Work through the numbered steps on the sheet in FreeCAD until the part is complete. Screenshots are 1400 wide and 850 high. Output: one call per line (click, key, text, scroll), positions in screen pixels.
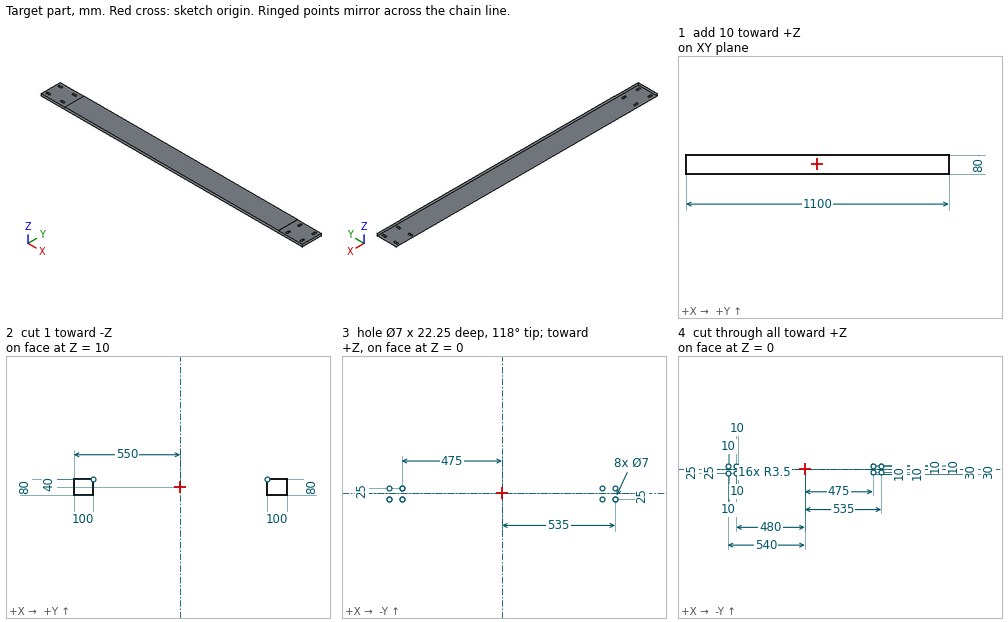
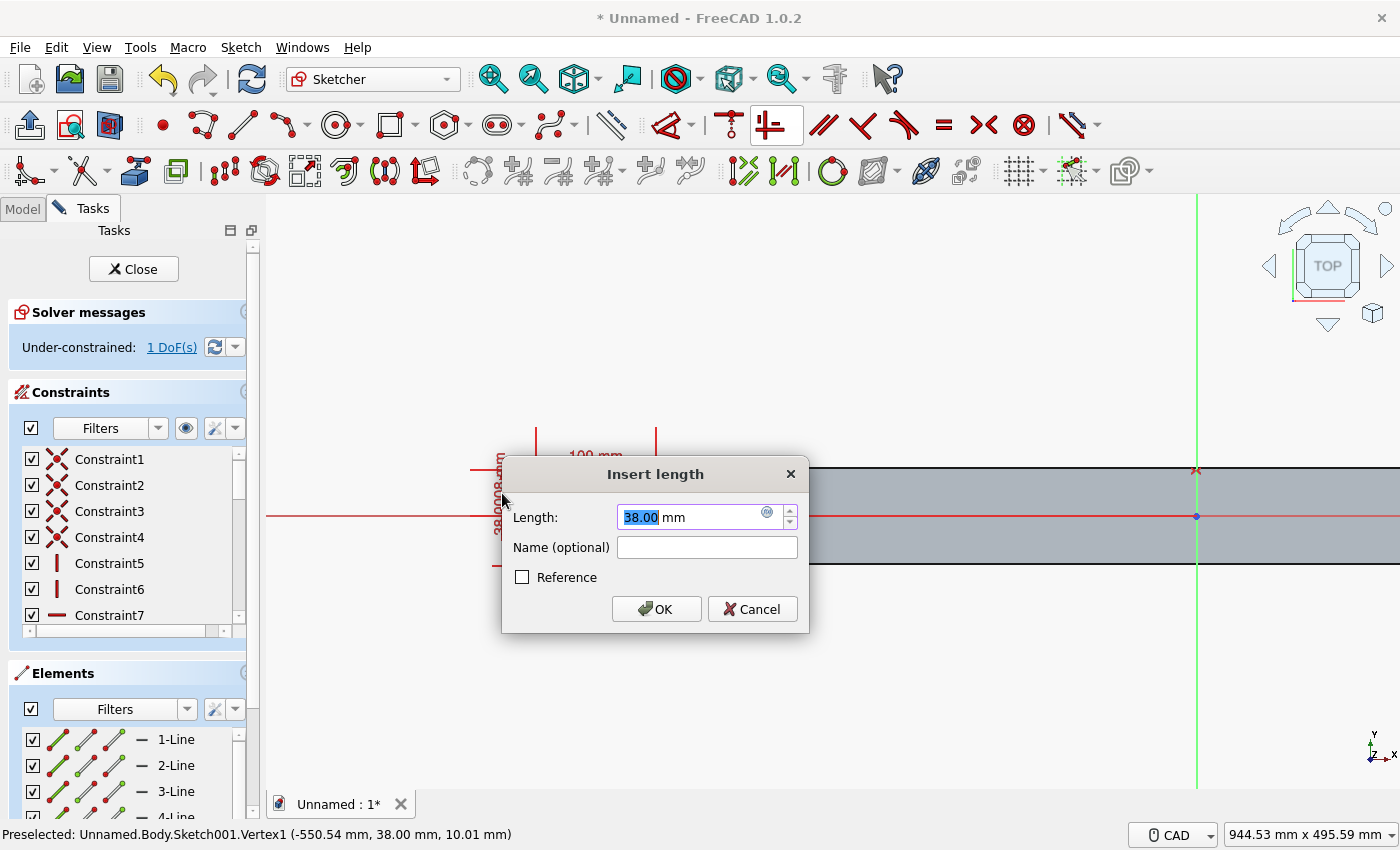
text(40)
key(Return)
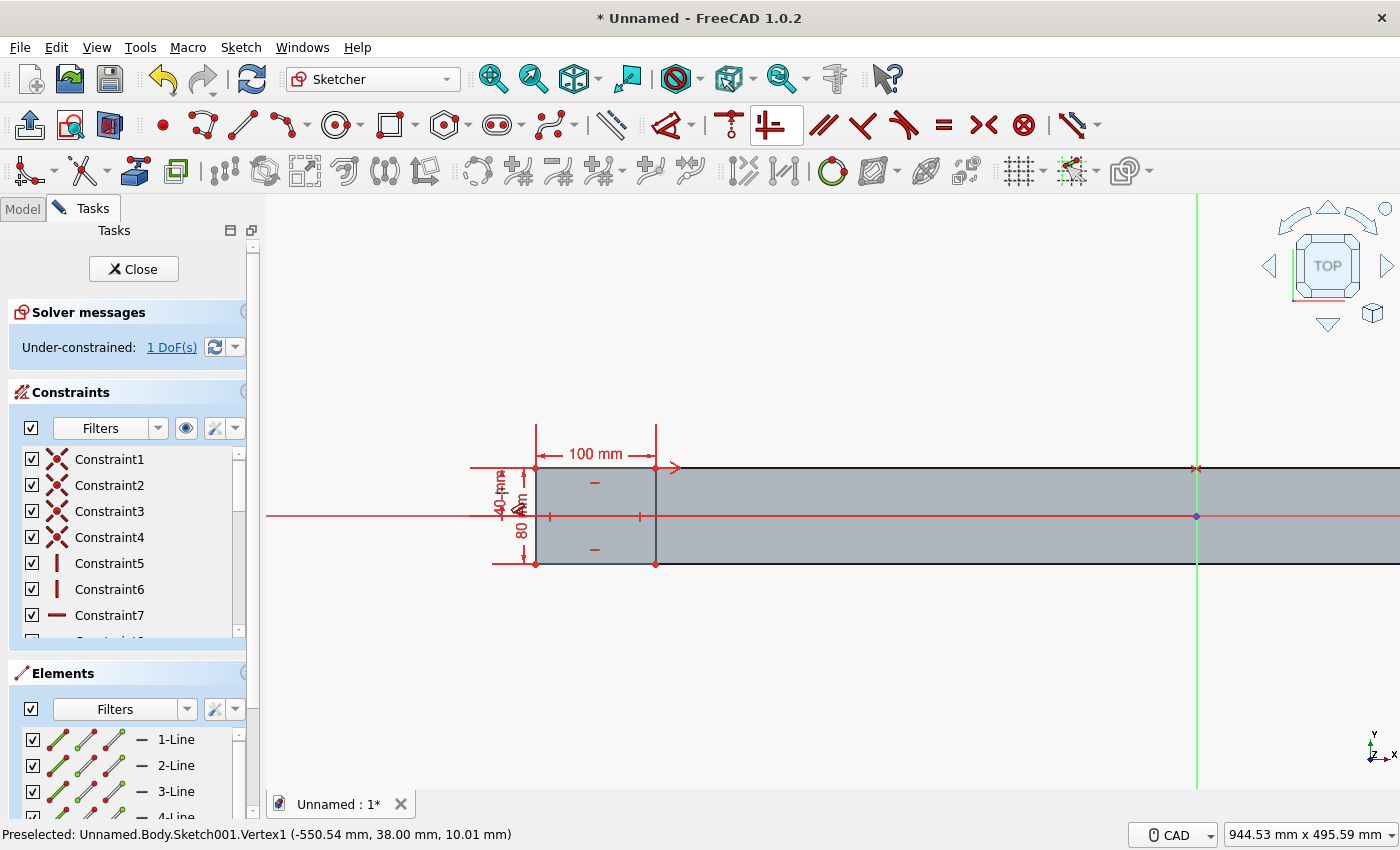
click(536, 468)
click(866, 434)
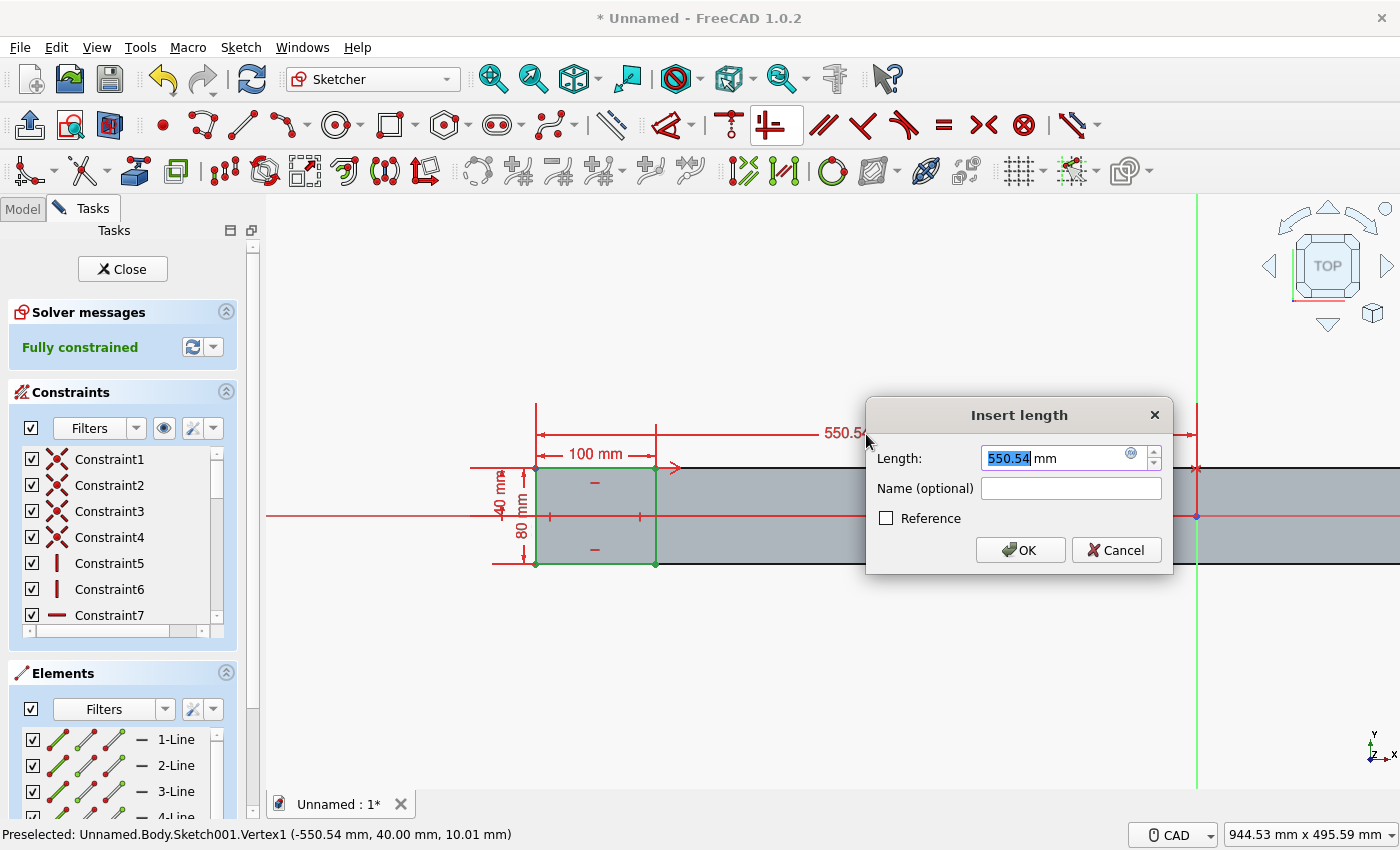
text(550)
key(Return)
key(Escape)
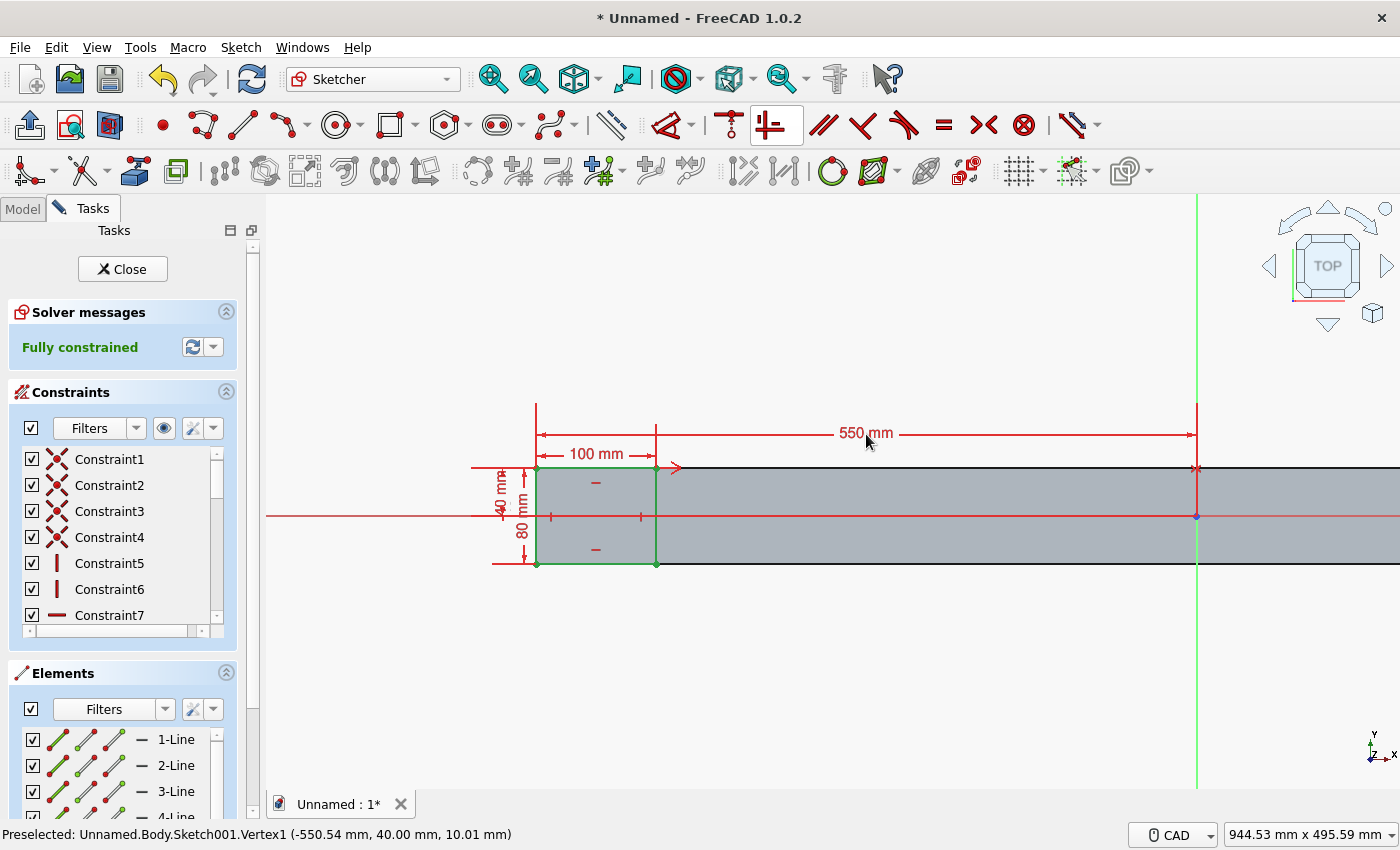
click(123, 269)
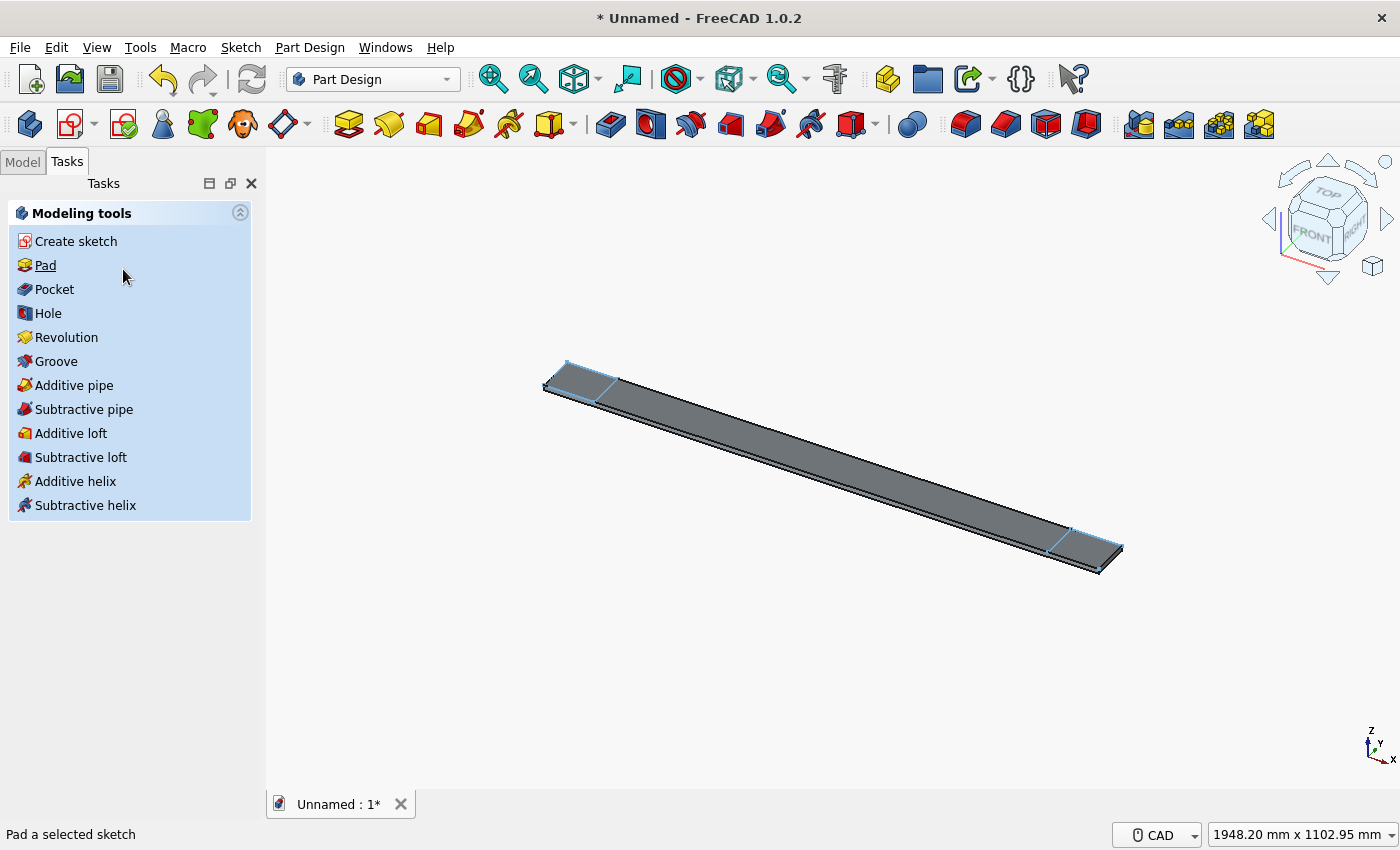
click(612, 124)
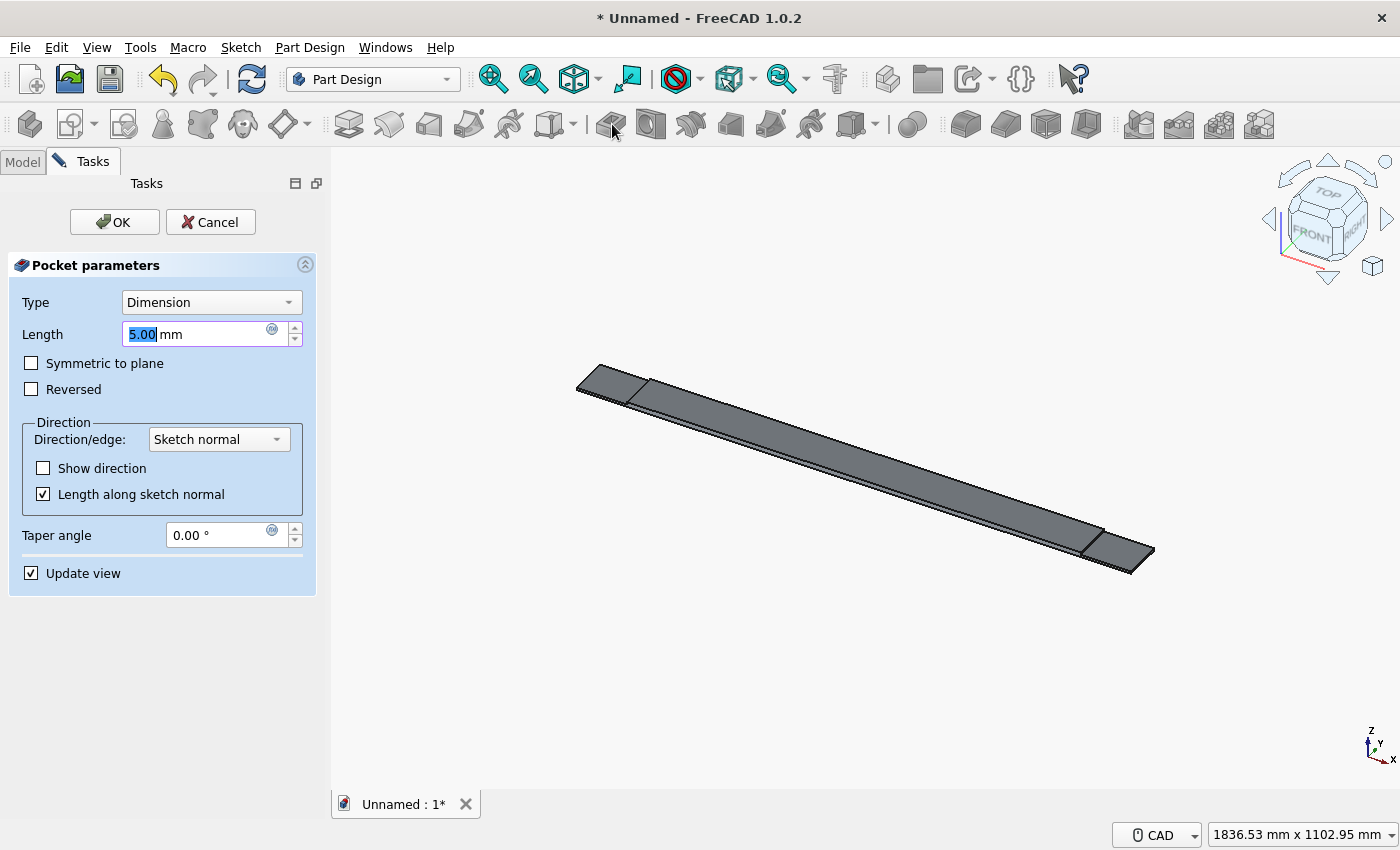
text(1)
key(Tab)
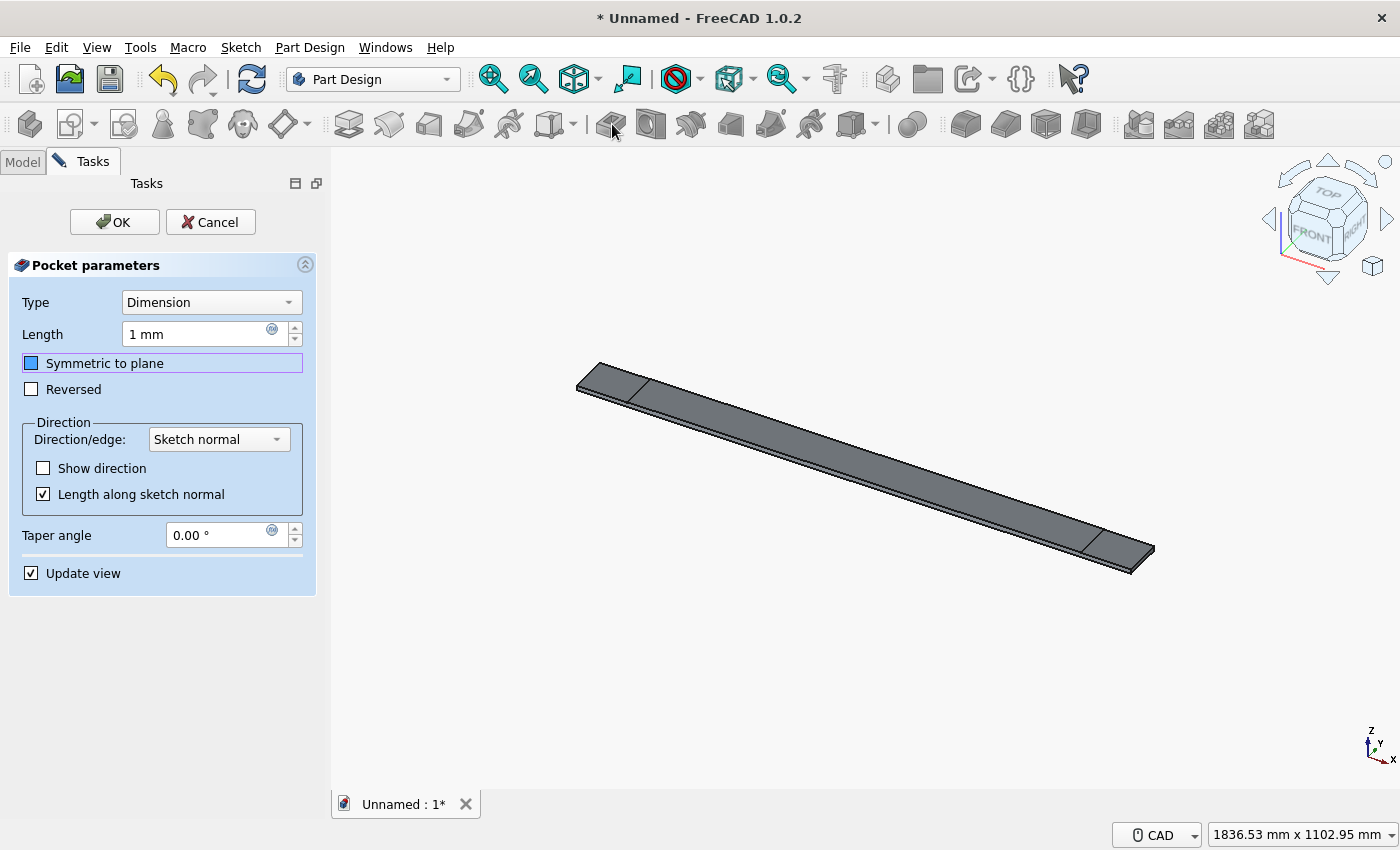
click(115, 222)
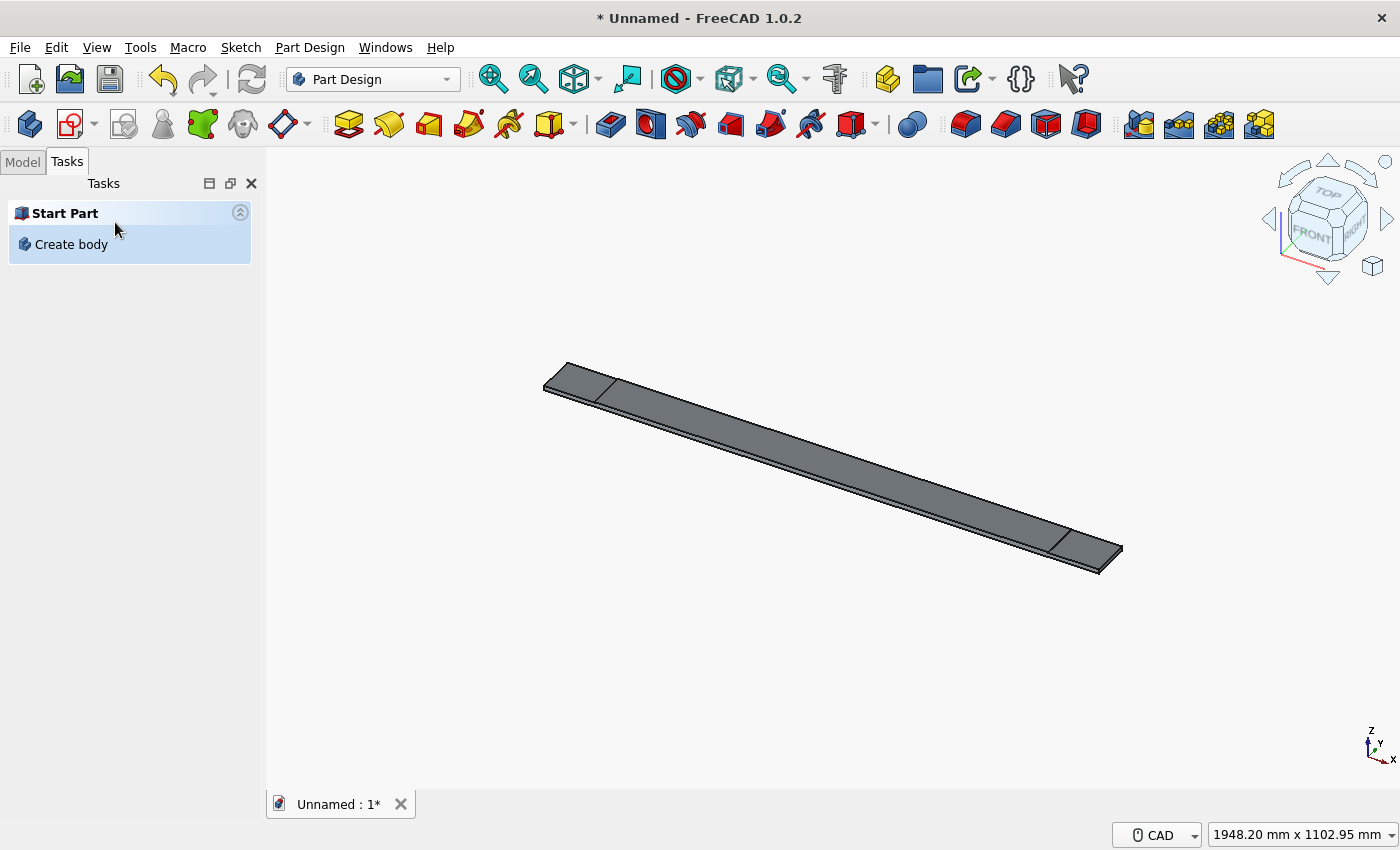
key(5)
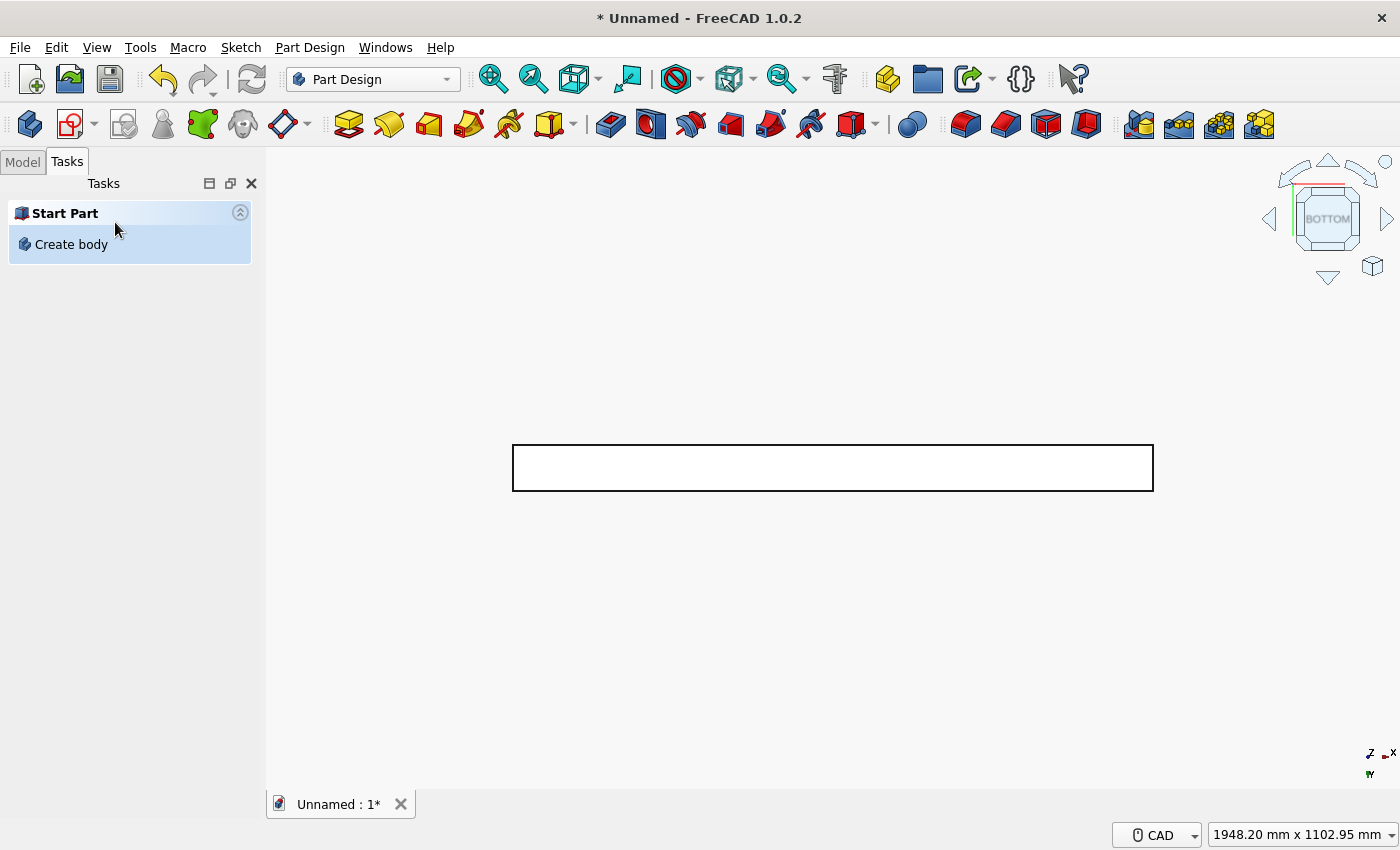
click(1107, 467)